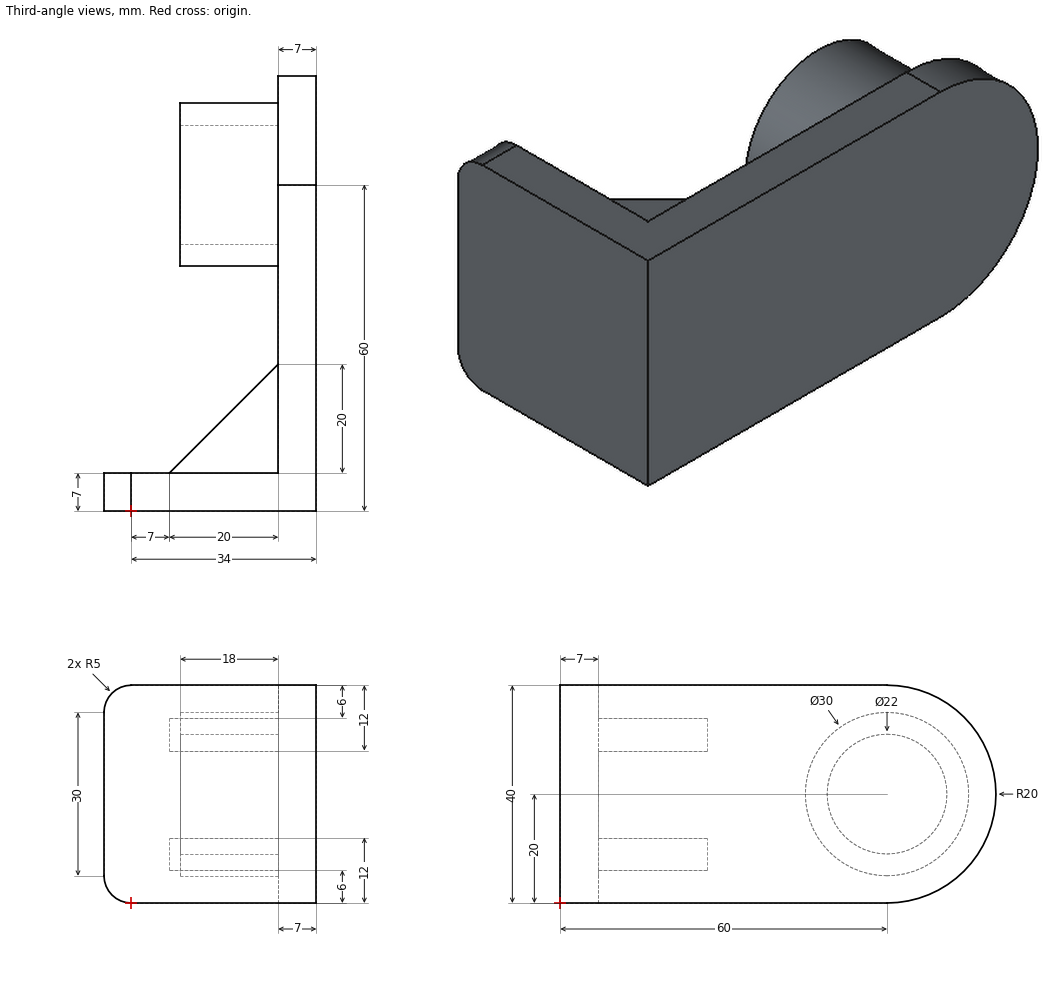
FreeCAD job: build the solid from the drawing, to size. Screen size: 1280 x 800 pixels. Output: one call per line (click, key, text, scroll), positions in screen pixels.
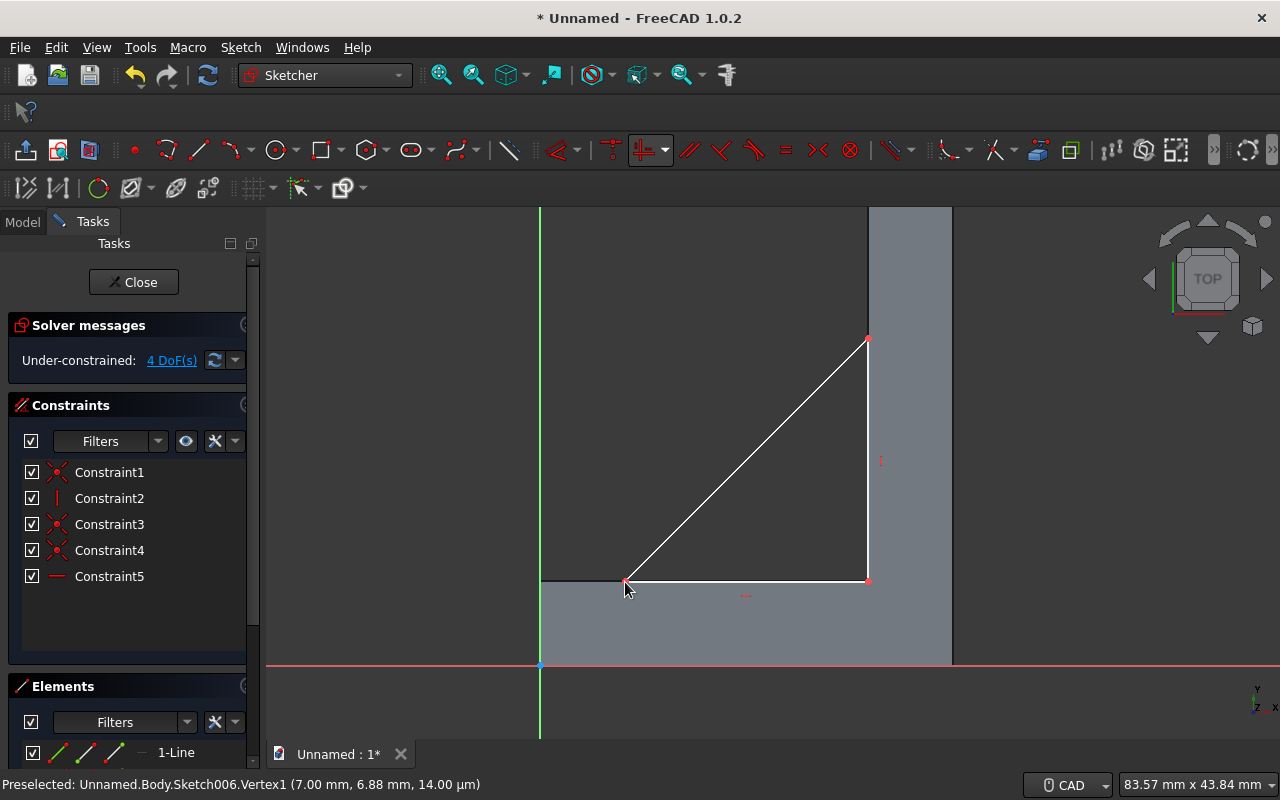
click(556, 150)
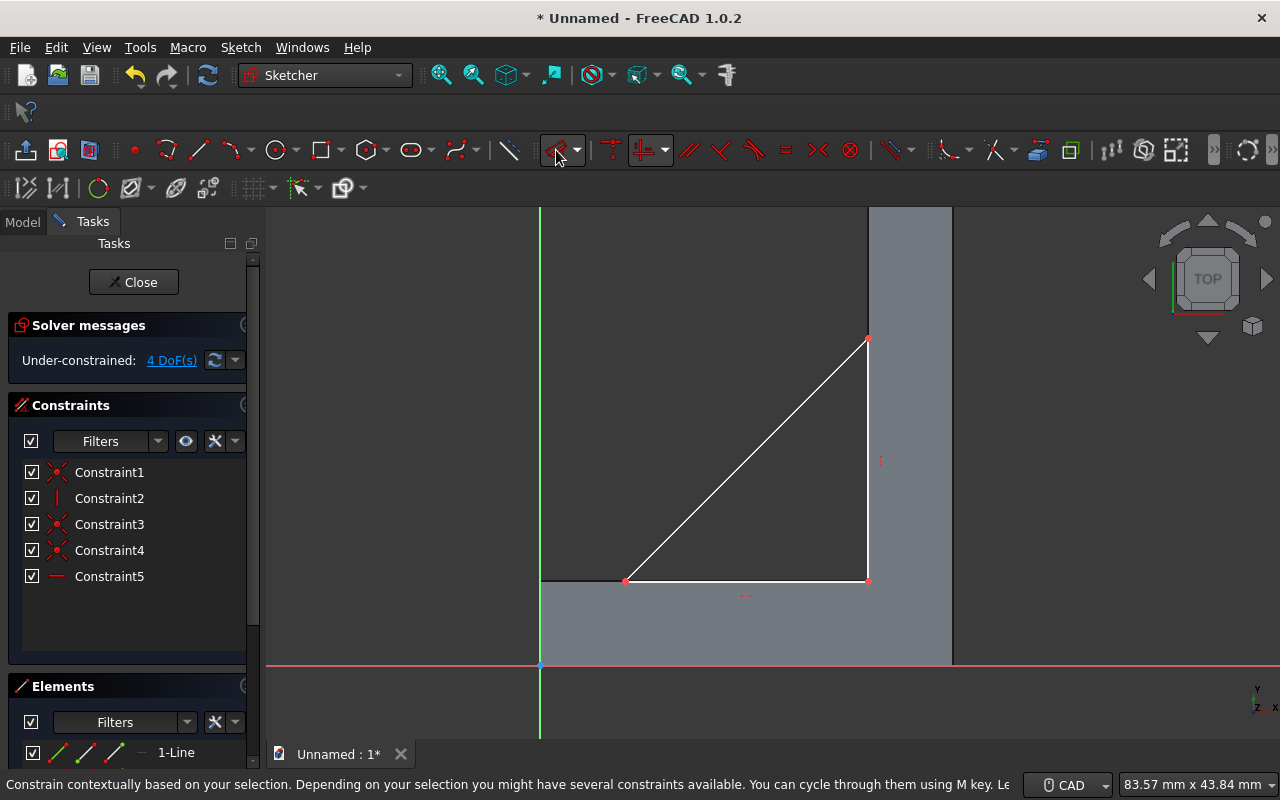
click(868, 412)
click(902, 461)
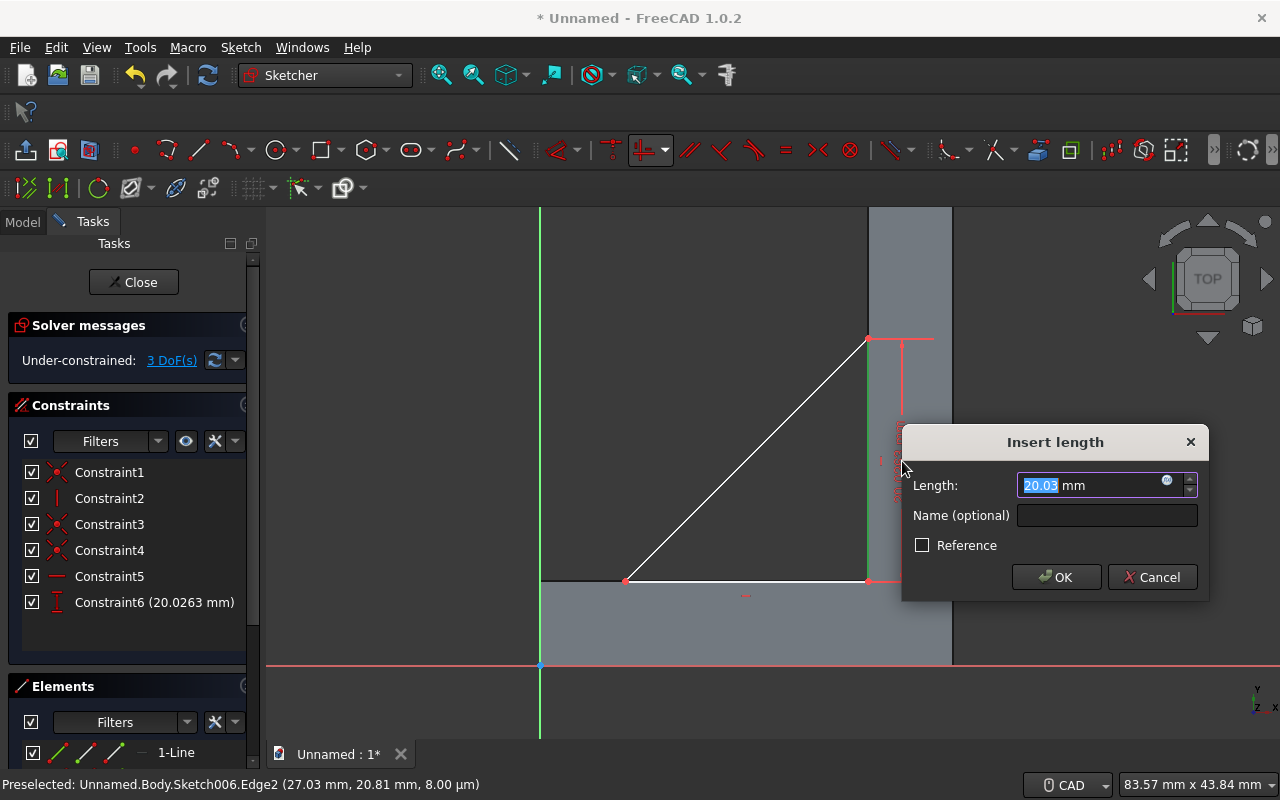
text(20)
key(Return)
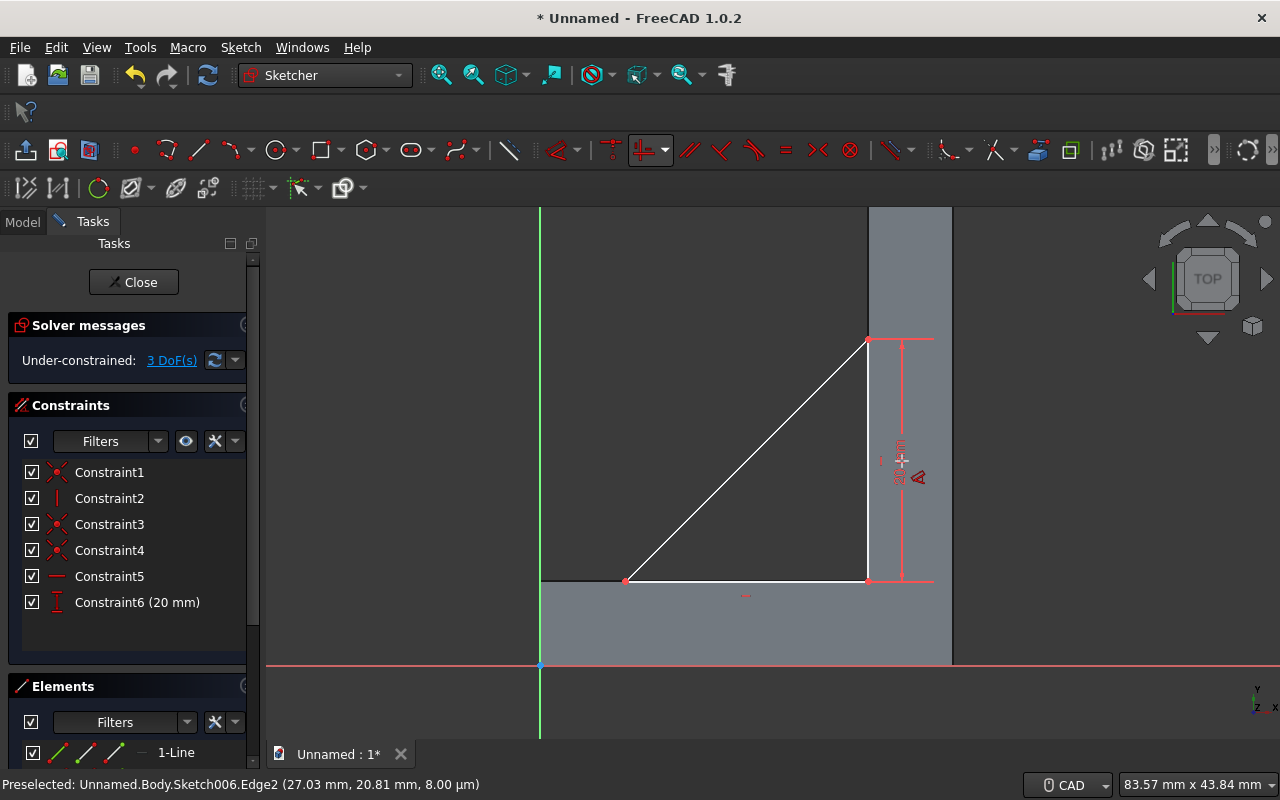
click(795, 582)
click(747, 616)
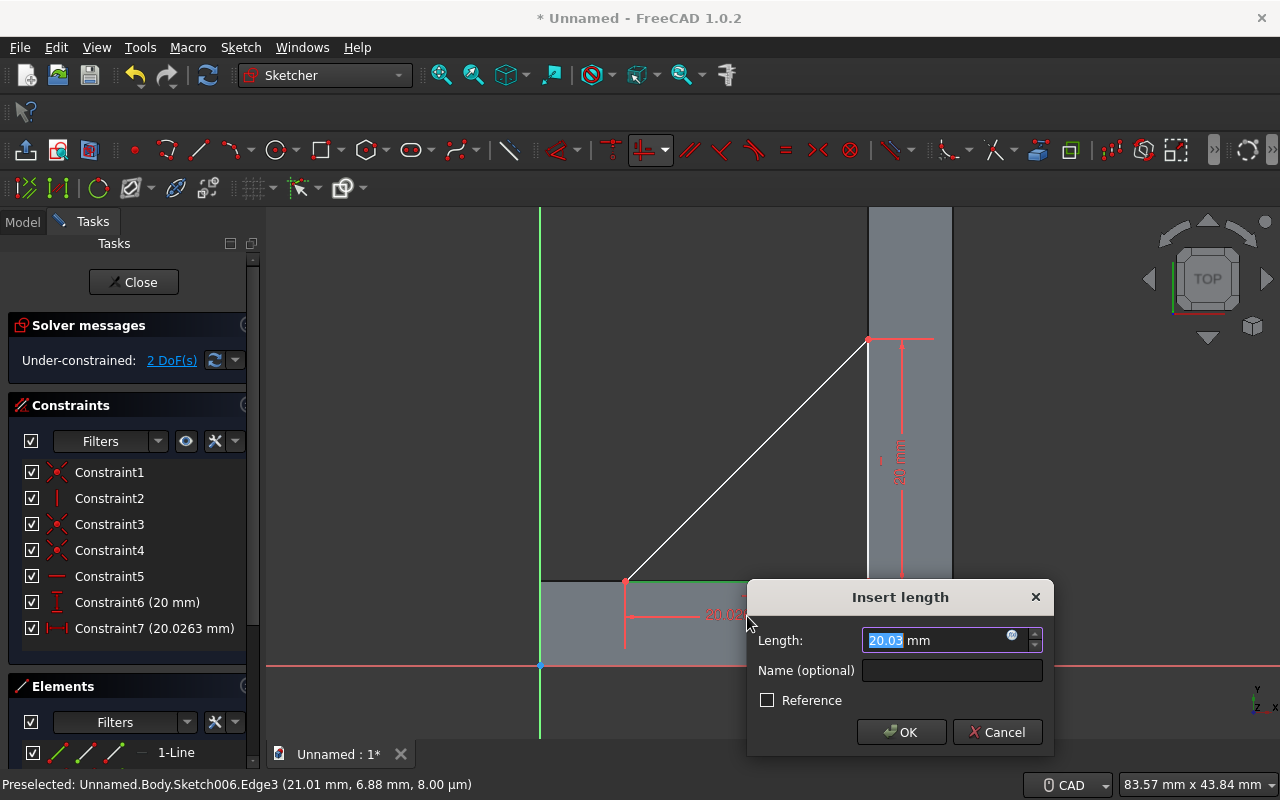
text(20)
key(Return)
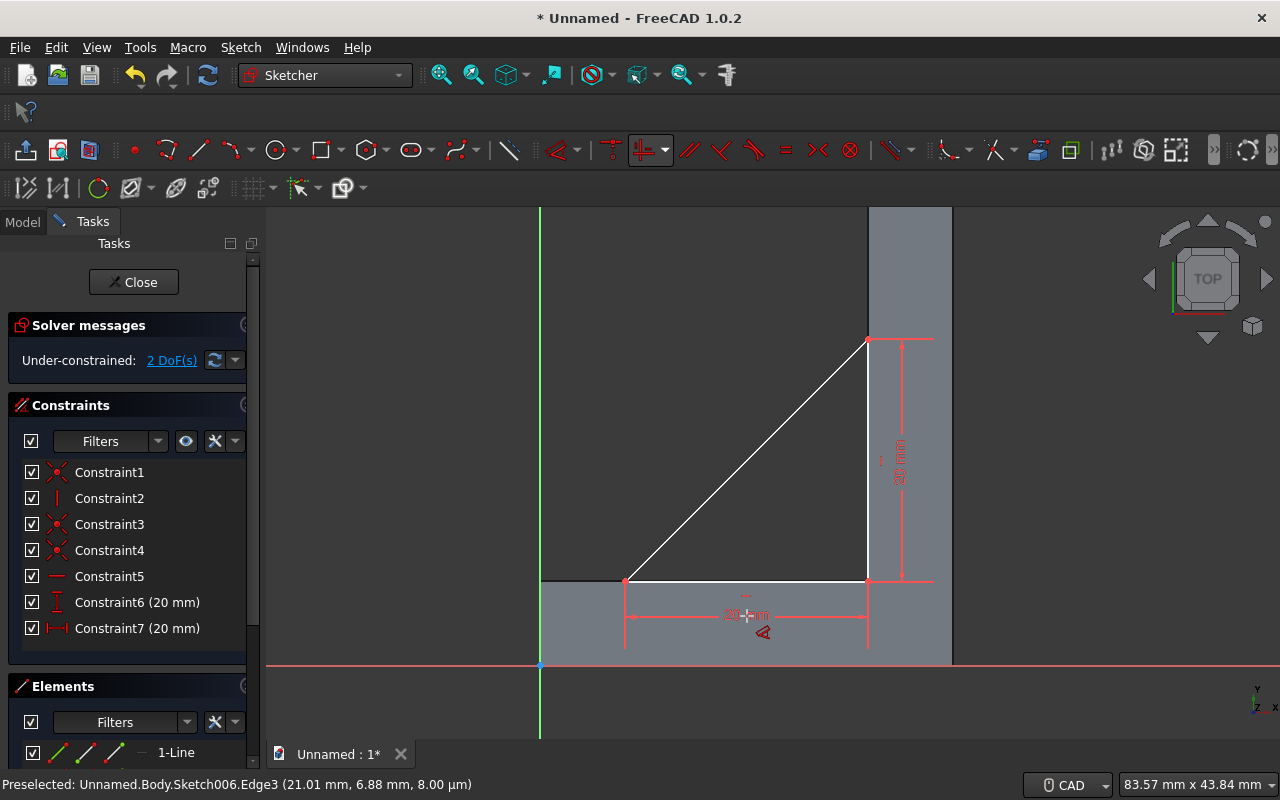
click(625, 582)
click(583, 700)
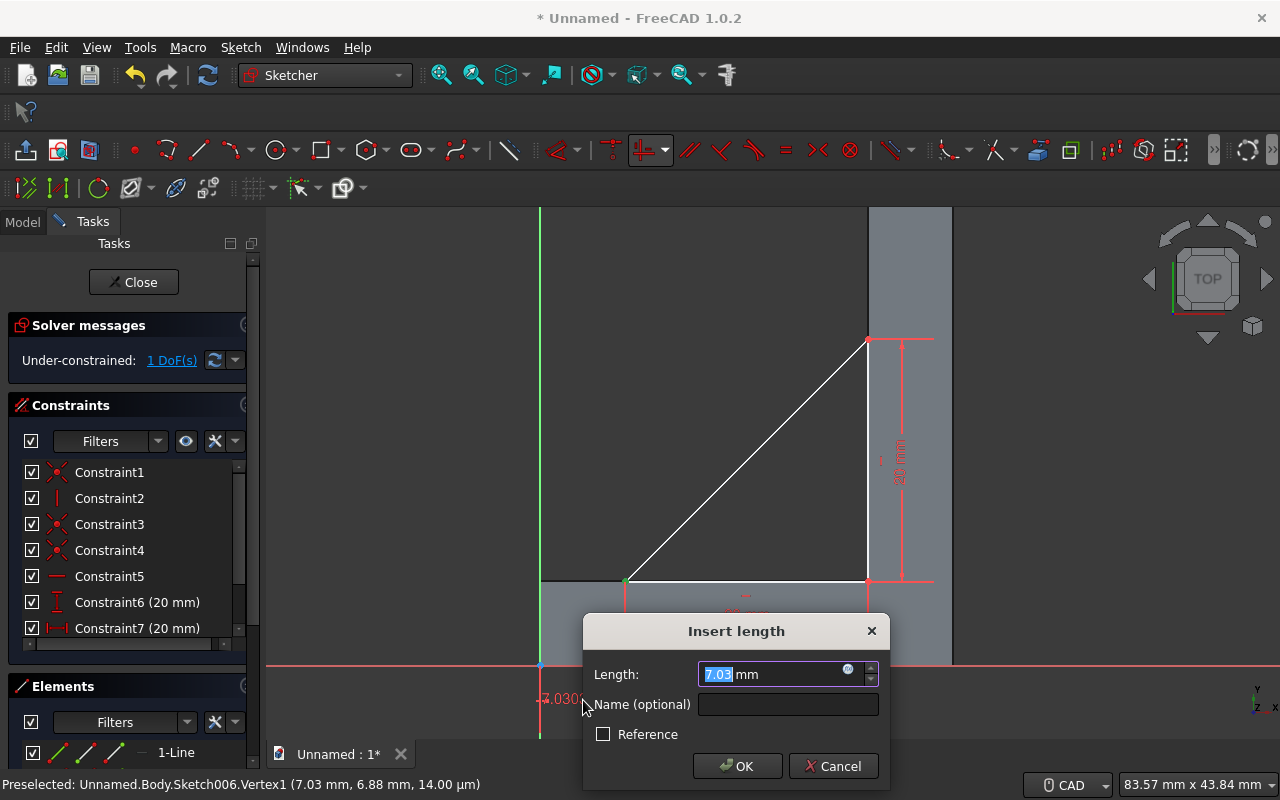
text(7)
key(Return)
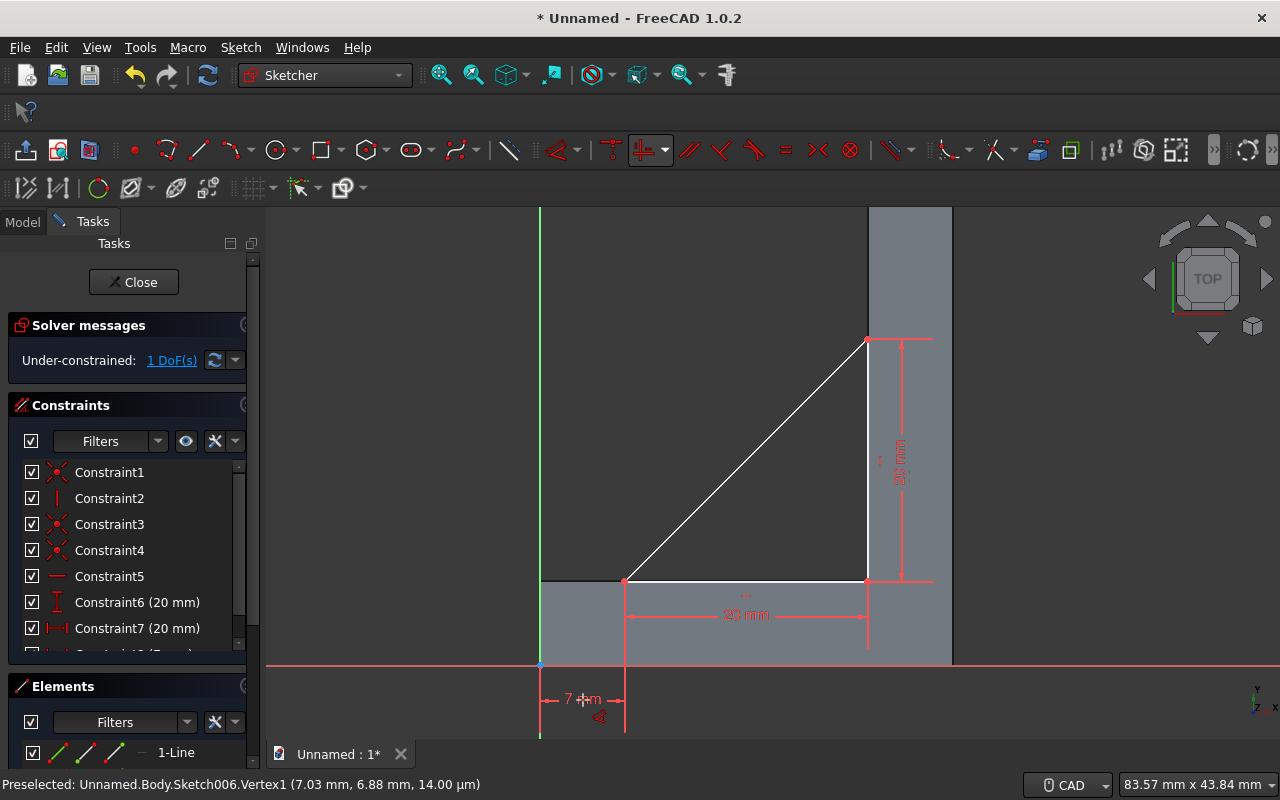
click(625, 582)
click(506, 624)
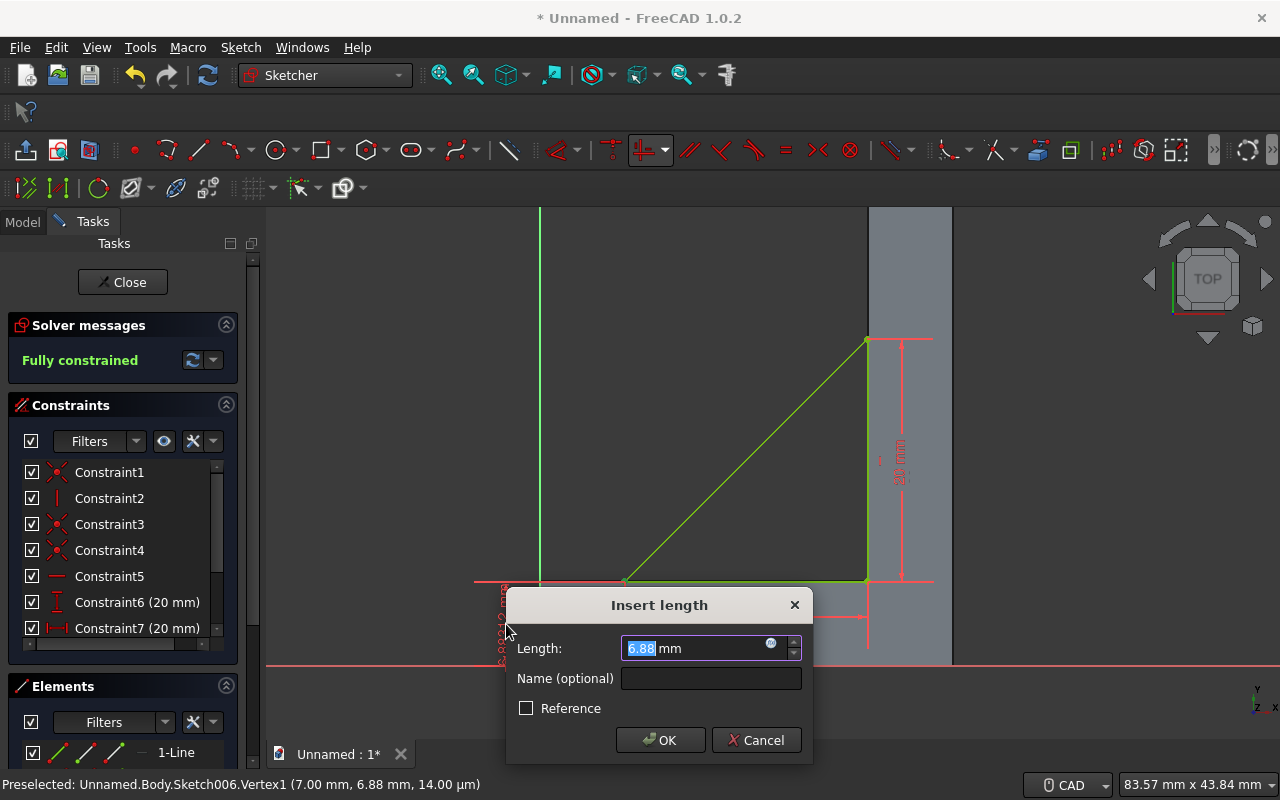
text(7)
key(Return)
key(Escape)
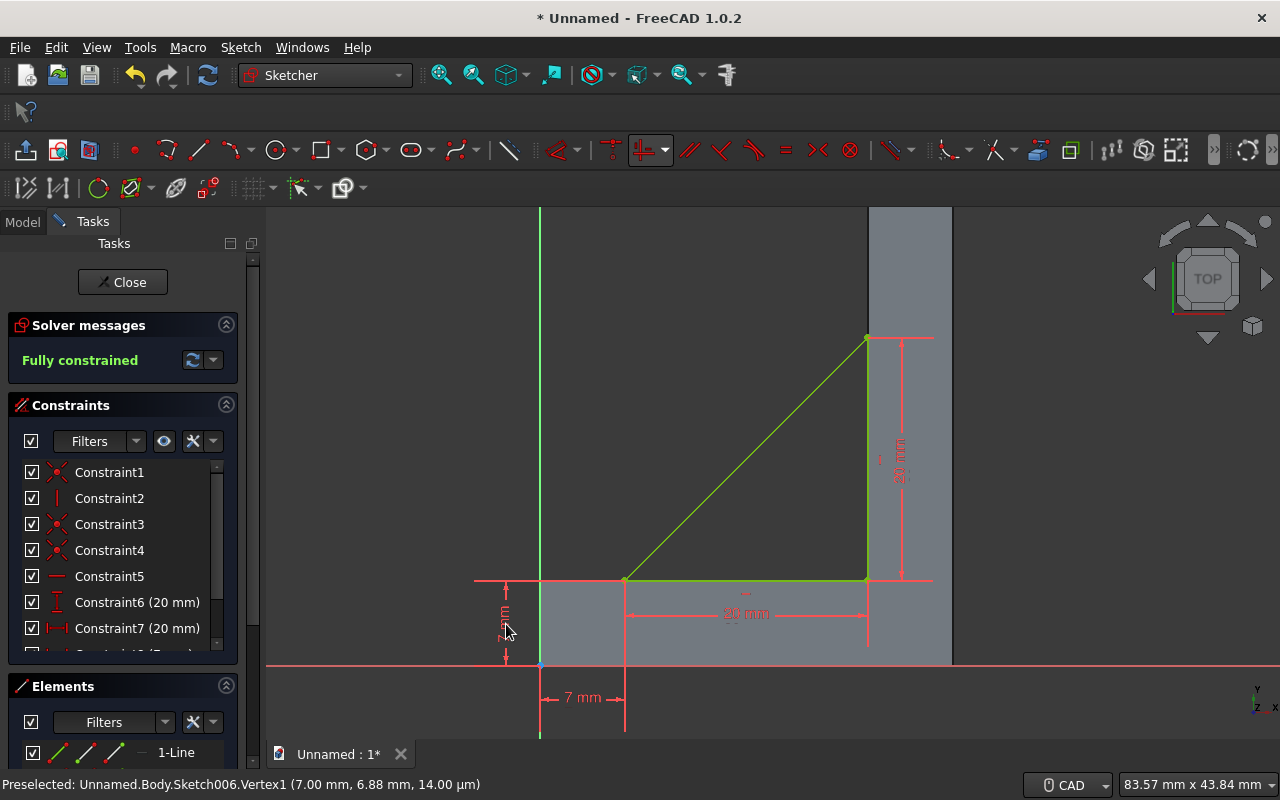
click(123, 282)